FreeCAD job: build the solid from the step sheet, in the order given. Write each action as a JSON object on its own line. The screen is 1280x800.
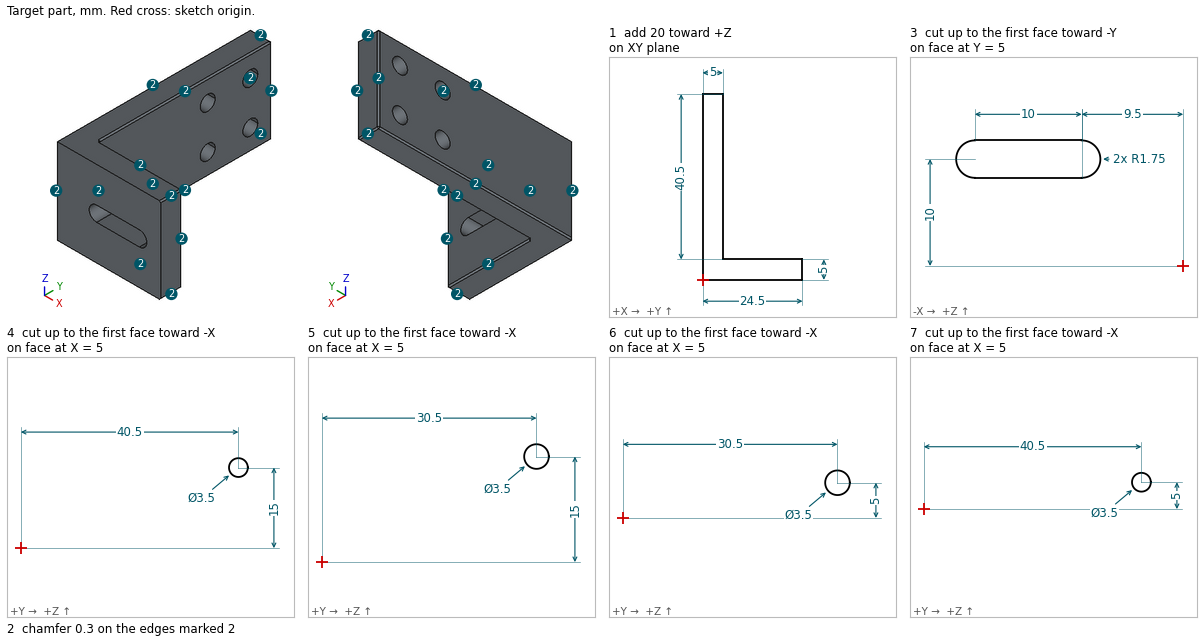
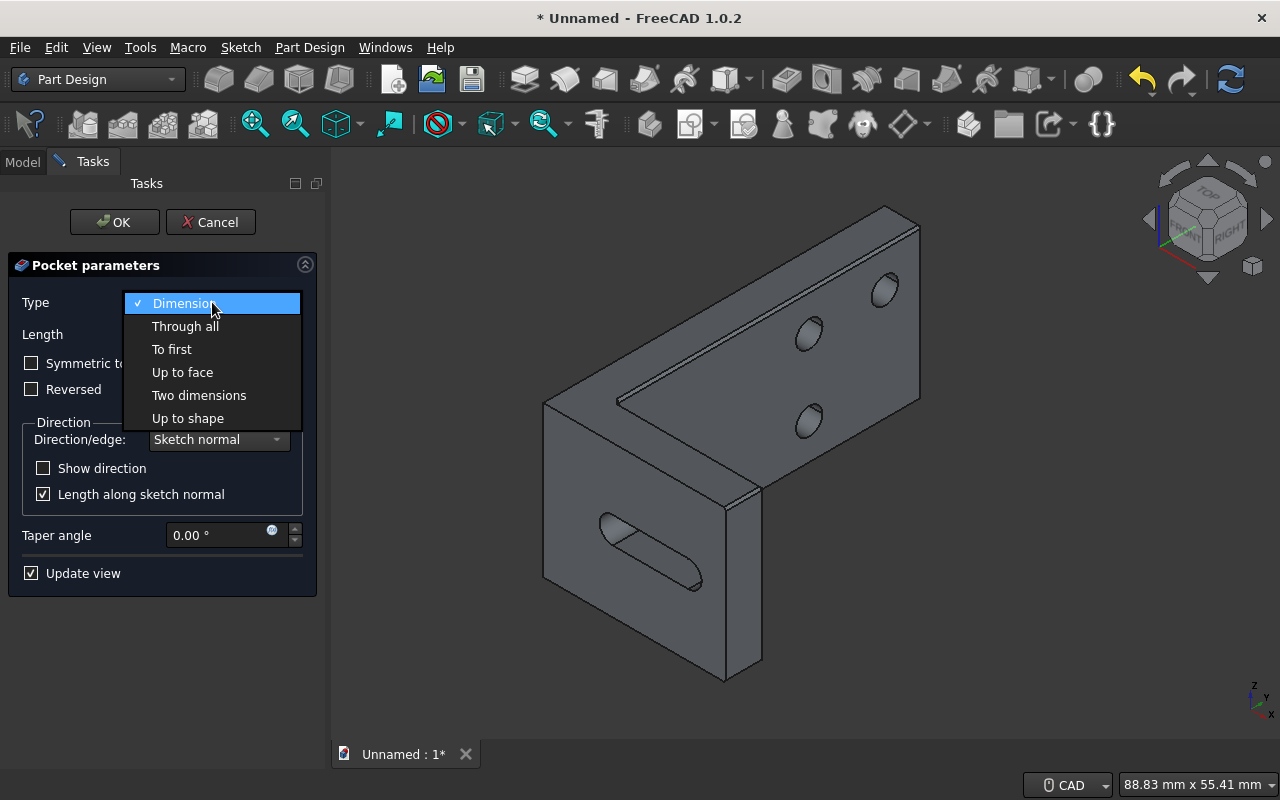
{"action": "left_click", "coordinate": [212, 350]}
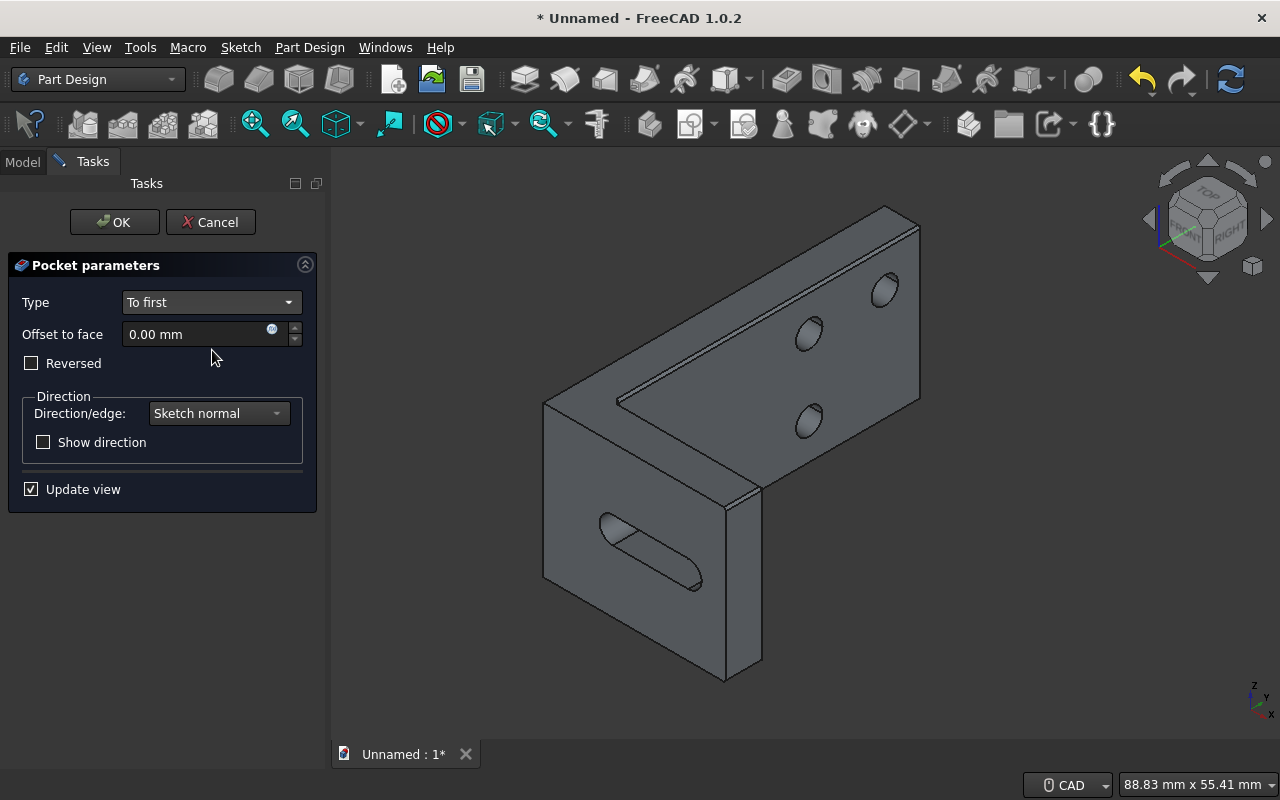
{"action": "left_click", "coordinate": [115, 222]}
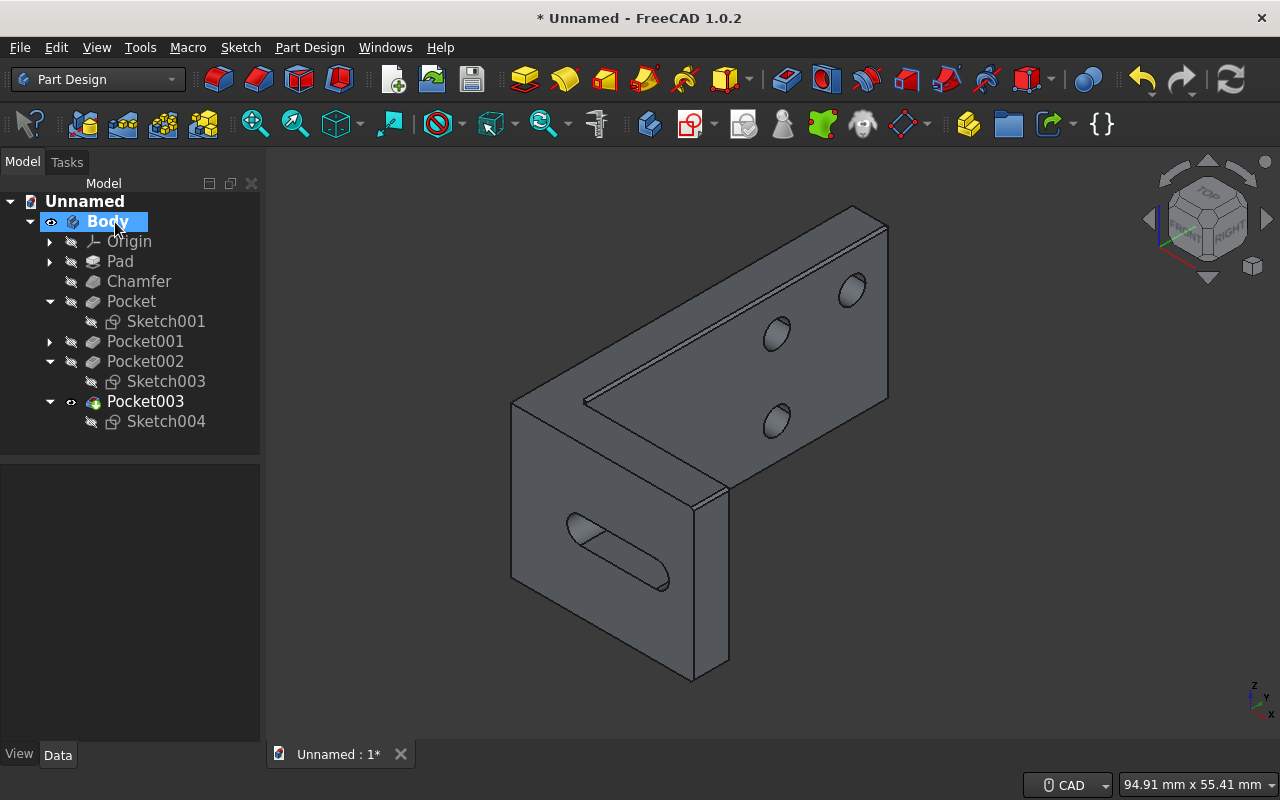
{"action": "left_click", "coordinate": [694, 424]}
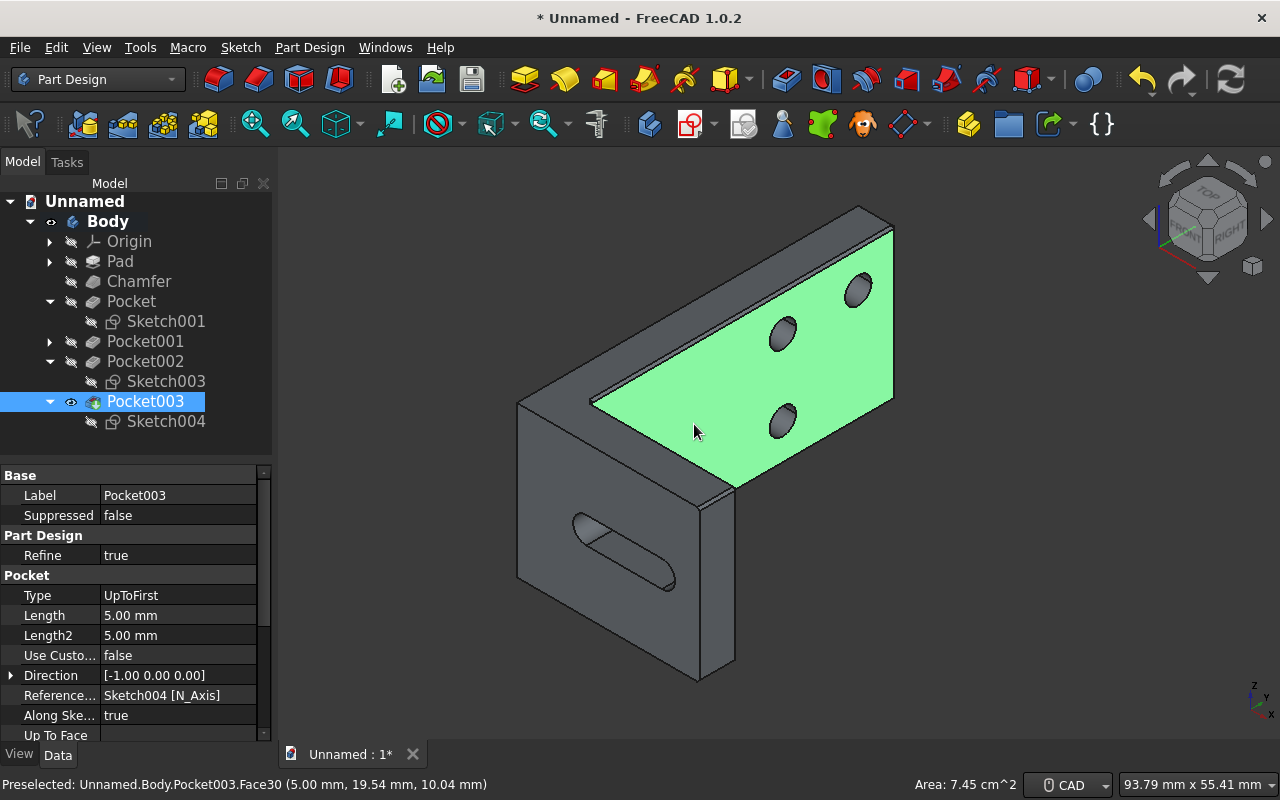
{"action": "left_click", "coordinate": [690, 124]}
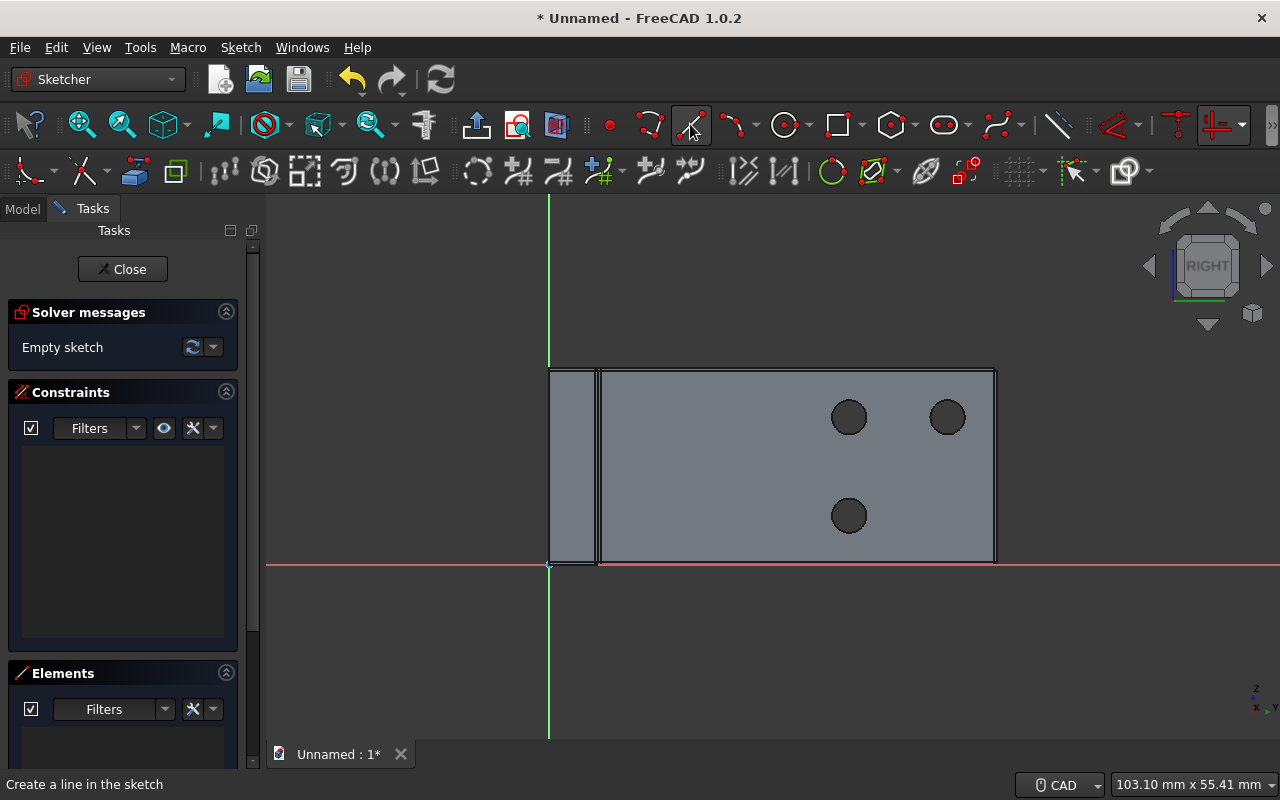
{"action": "left_click", "coordinate": [558, 126]}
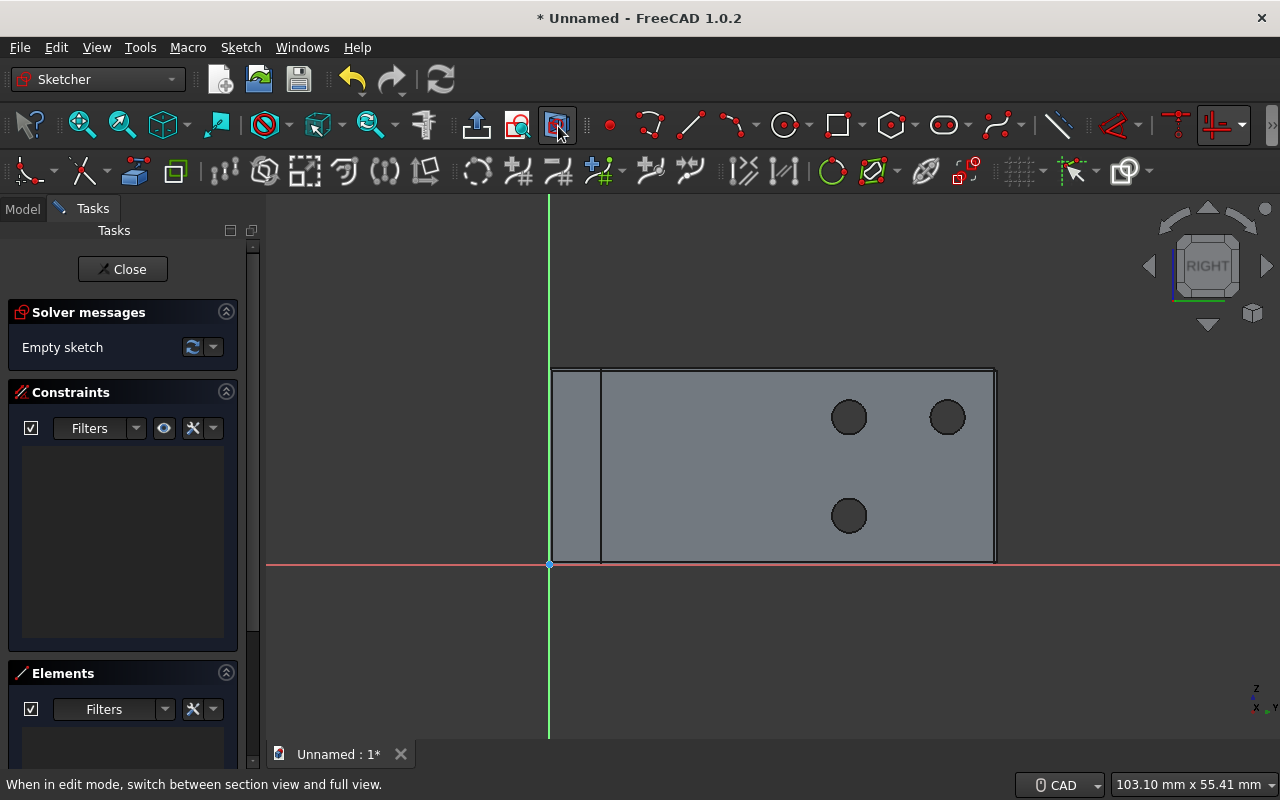
{"action": "scroll", "coordinate": [972, 521], "scroll_direction": "up", "scroll_amount": 12}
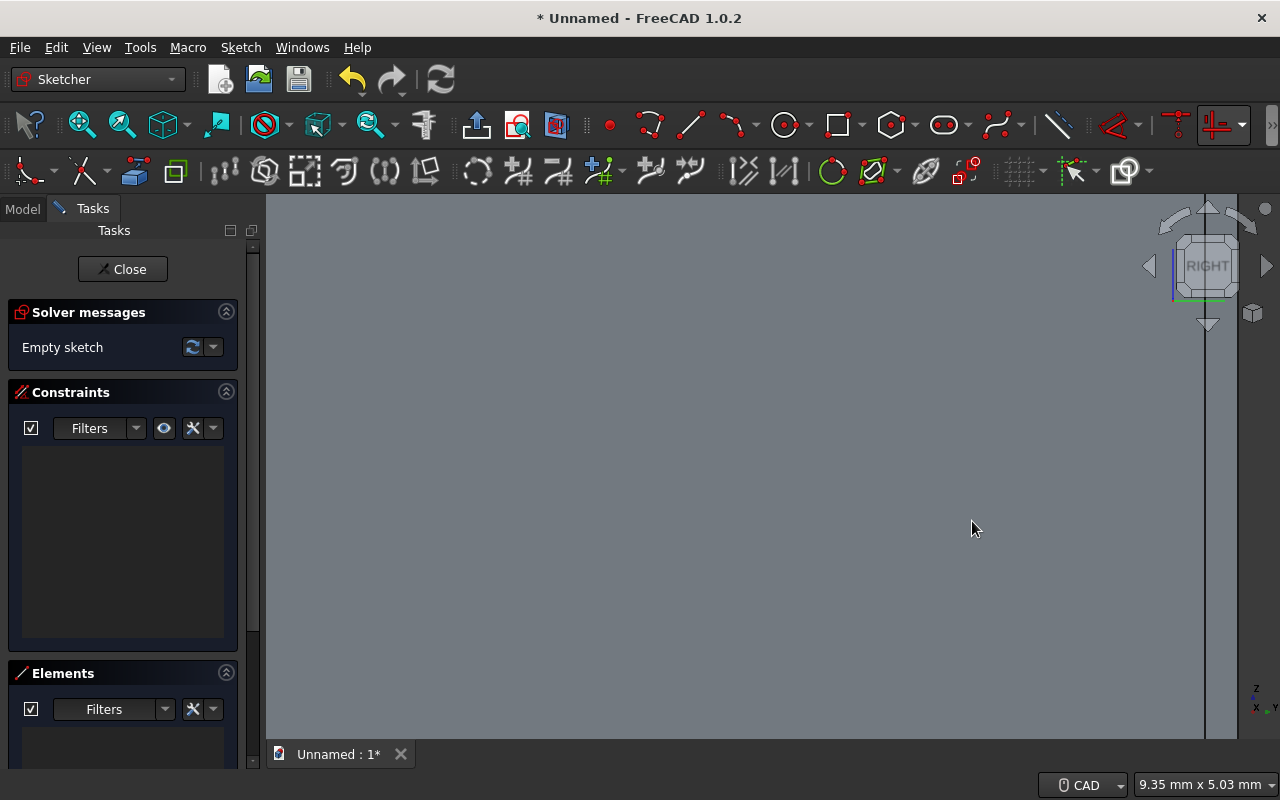
{"action": "left_click", "coordinate": [786, 126]}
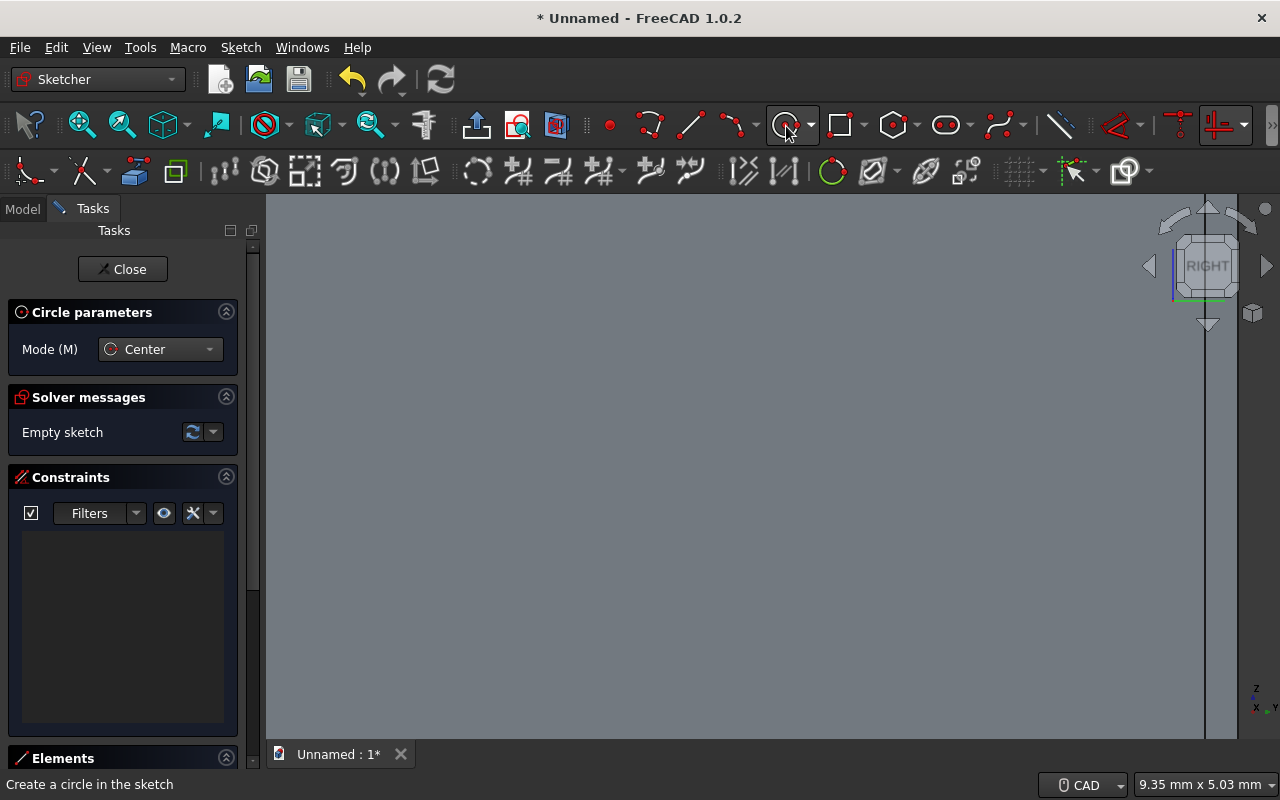
{"action": "left_click", "coordinate": [696, 456]}
{"action": "left_click", "coordinate": [830, 322]}
{"action": "key", "text": "Escape"}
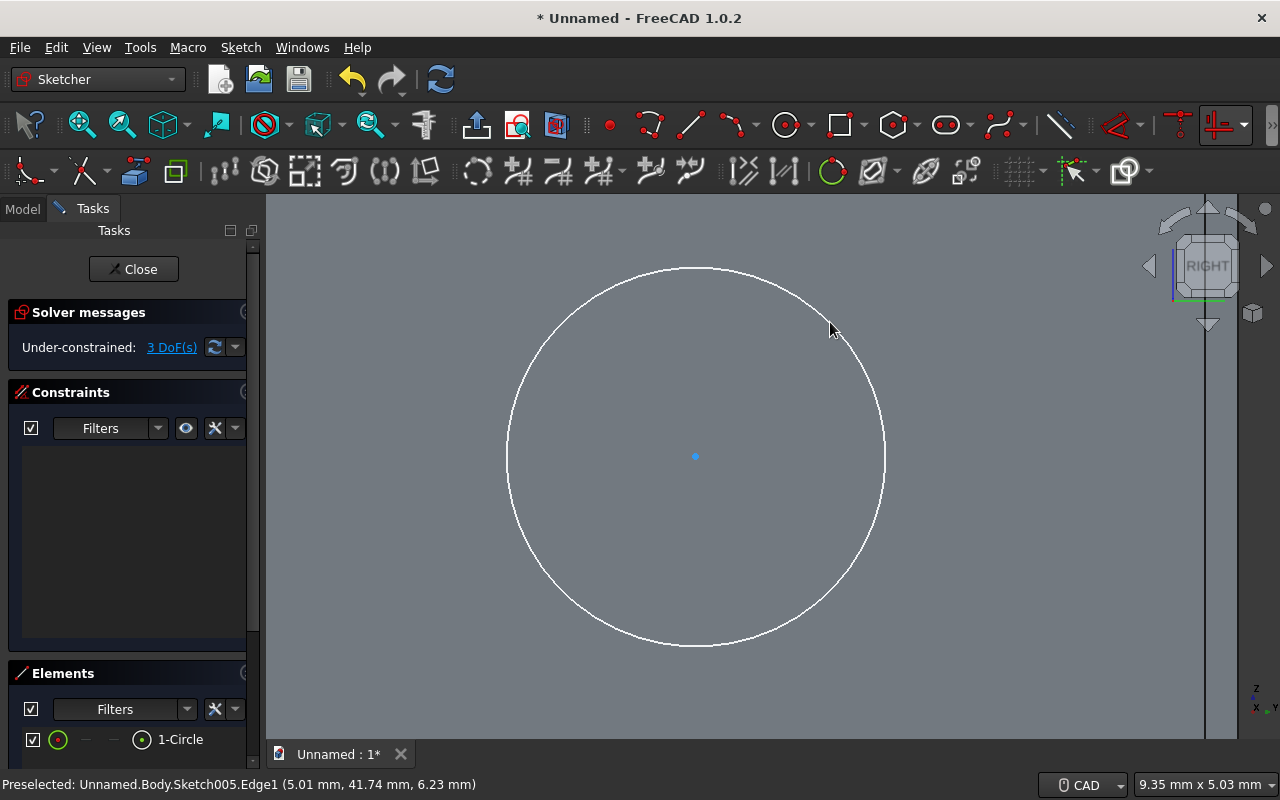
{"action": "left_click", "coordinate": [1116, 126]}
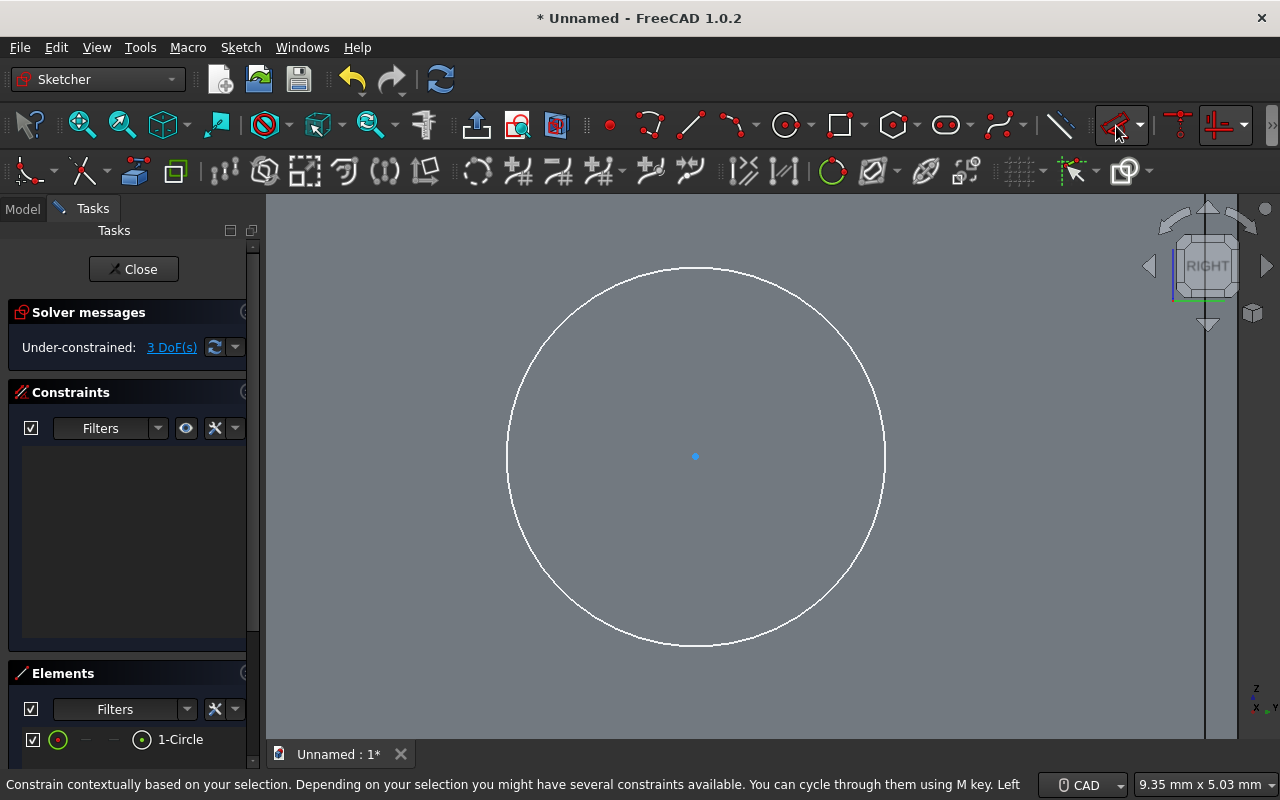
{"action": "left_click", "coordinate": [830, 323]}
{"action": "left_click", "coordinate": [853, 300]}